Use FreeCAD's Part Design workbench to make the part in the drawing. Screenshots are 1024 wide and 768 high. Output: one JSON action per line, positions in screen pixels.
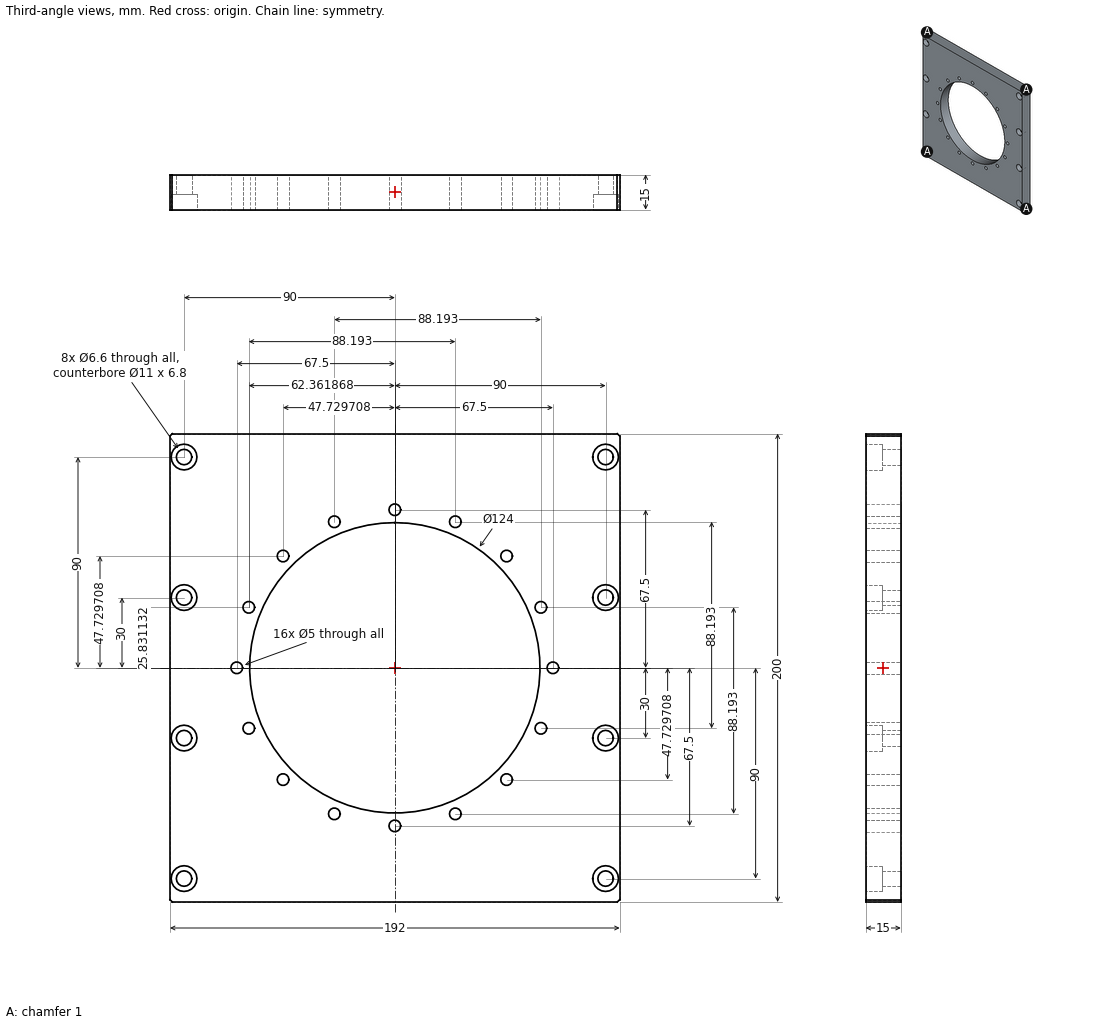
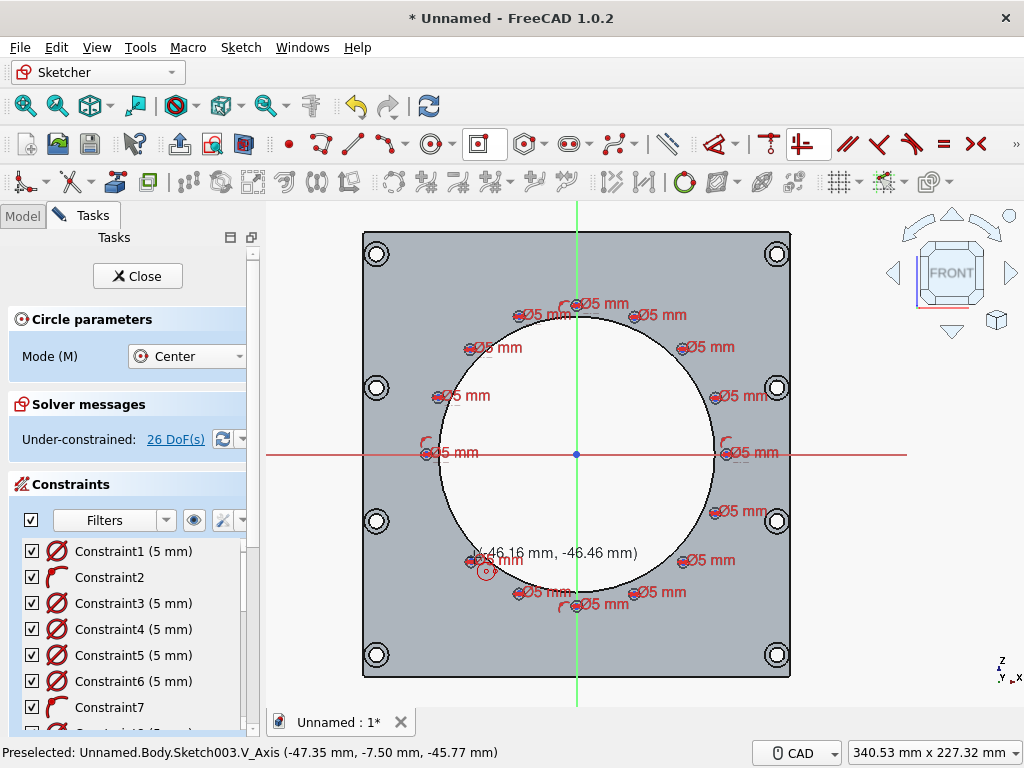
{"action": "scroll", "coordinate": [438, 512], "scroll_direction": "up", "scroll_amount": 8}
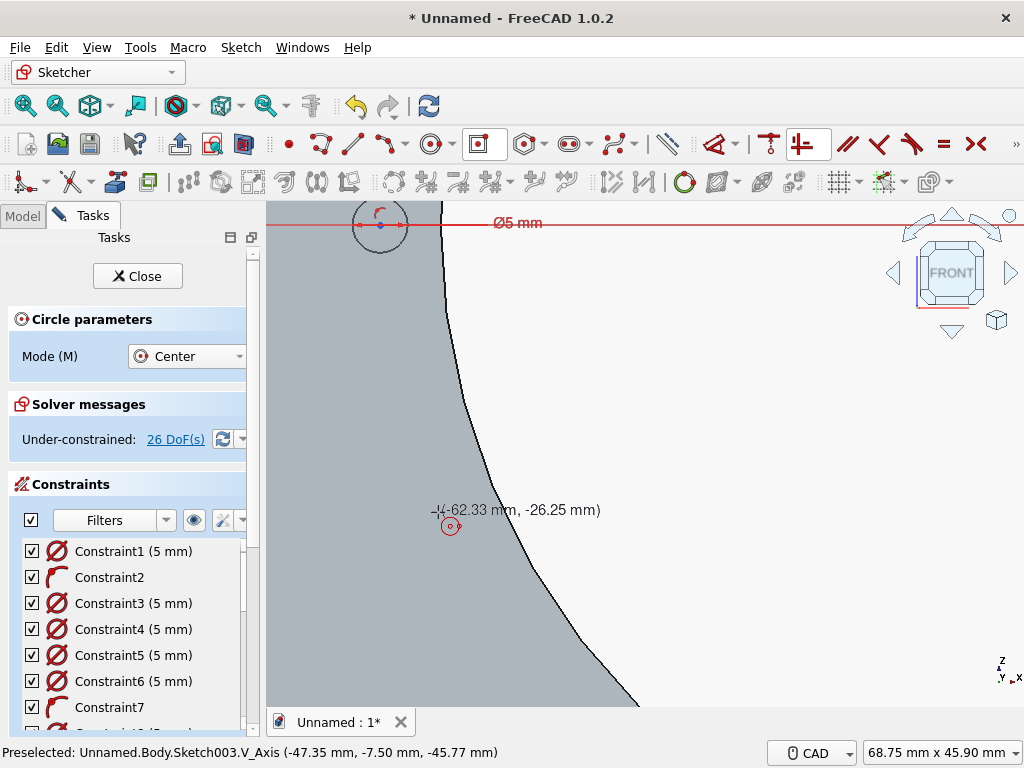
{"action": "scroll", "coordinate": [438, 512], "scroll_direction": "down", "scroll_amount": 8}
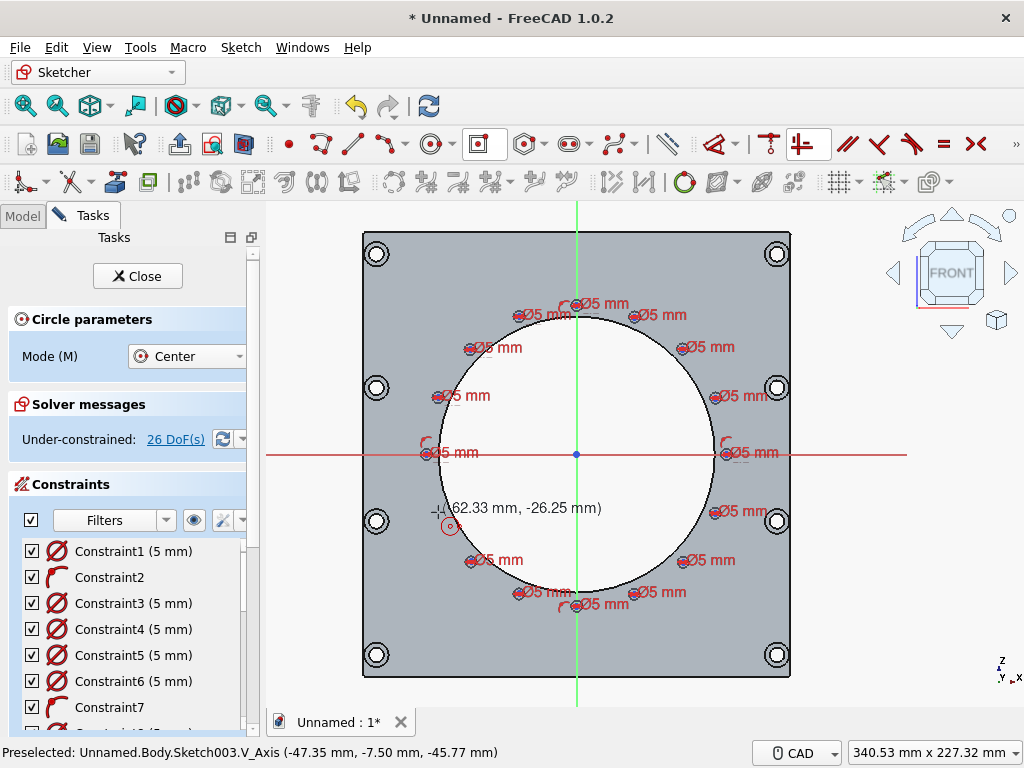
{"action": "left_click", "coordinate": [438, 512]}
{"action": "mouse_move", "coordinate": [442, 508]}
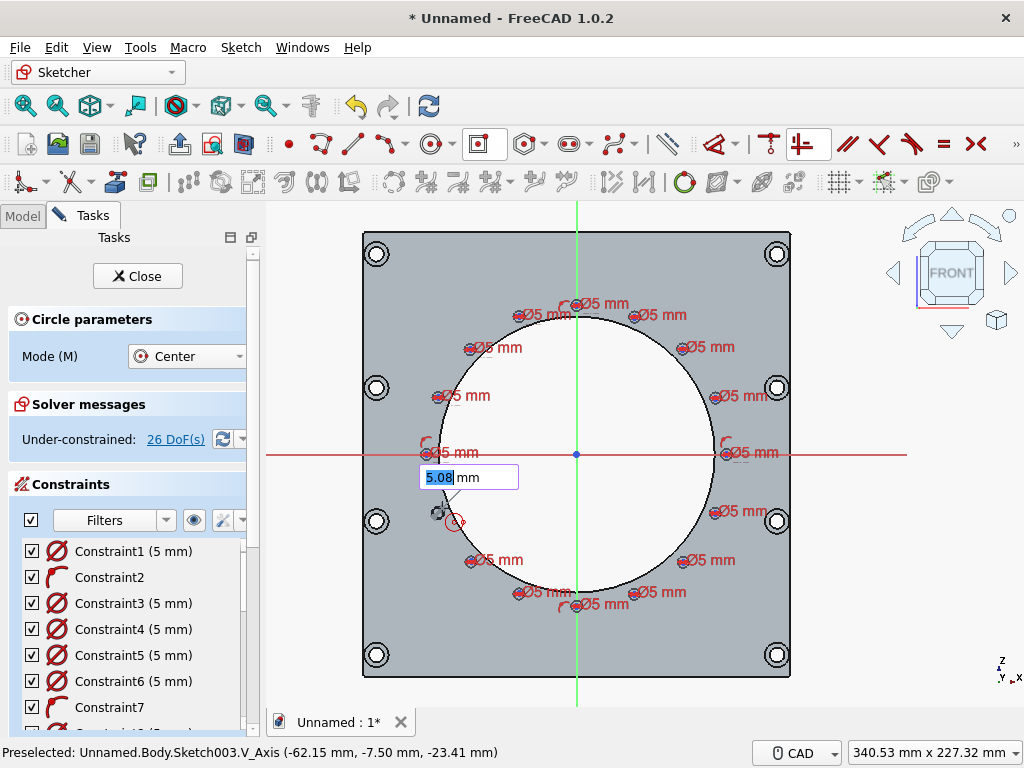
{"action": "type", "text": "5"}
{"action": "key", "text": "Return"}
{"action": "key", "text": "Escape"}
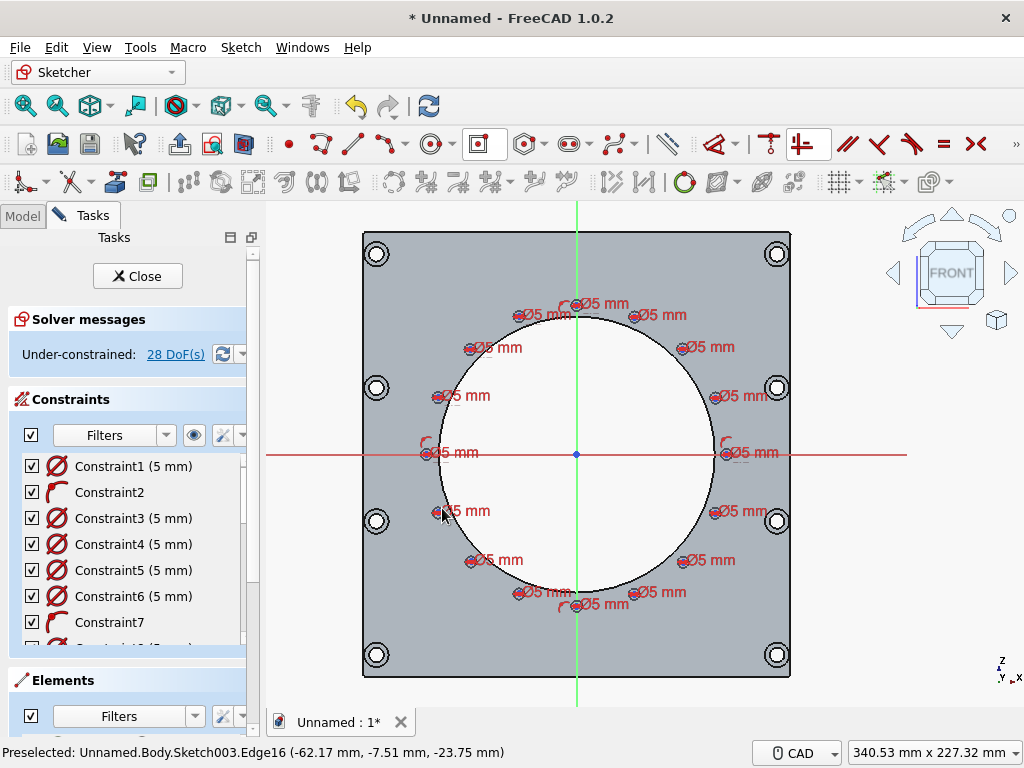
{"action": "left_click", "coordinate": [519, 317]}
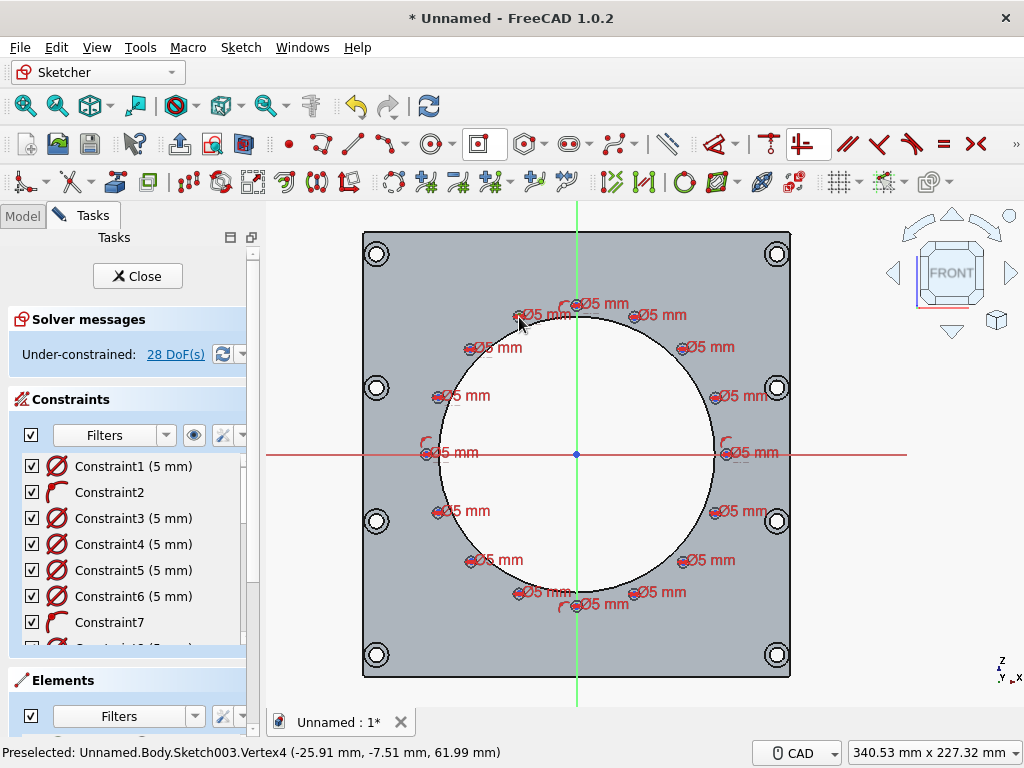
{"action": "left_click", "coordinate": [635, 317]}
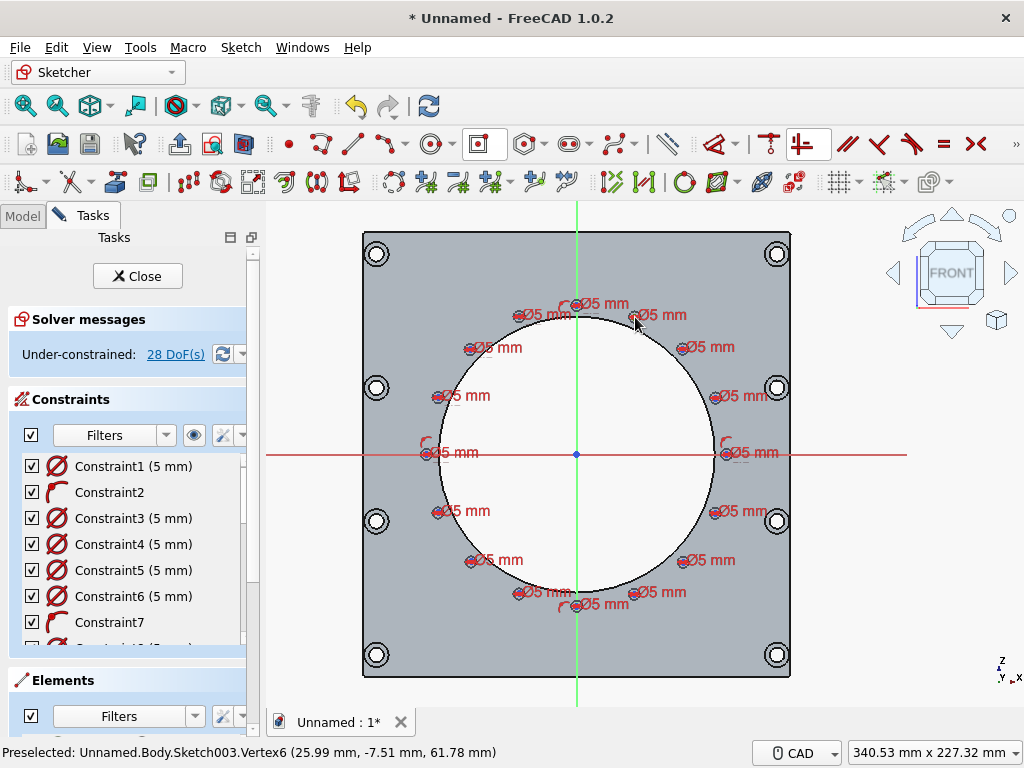
{"action": "key", "text": "h"}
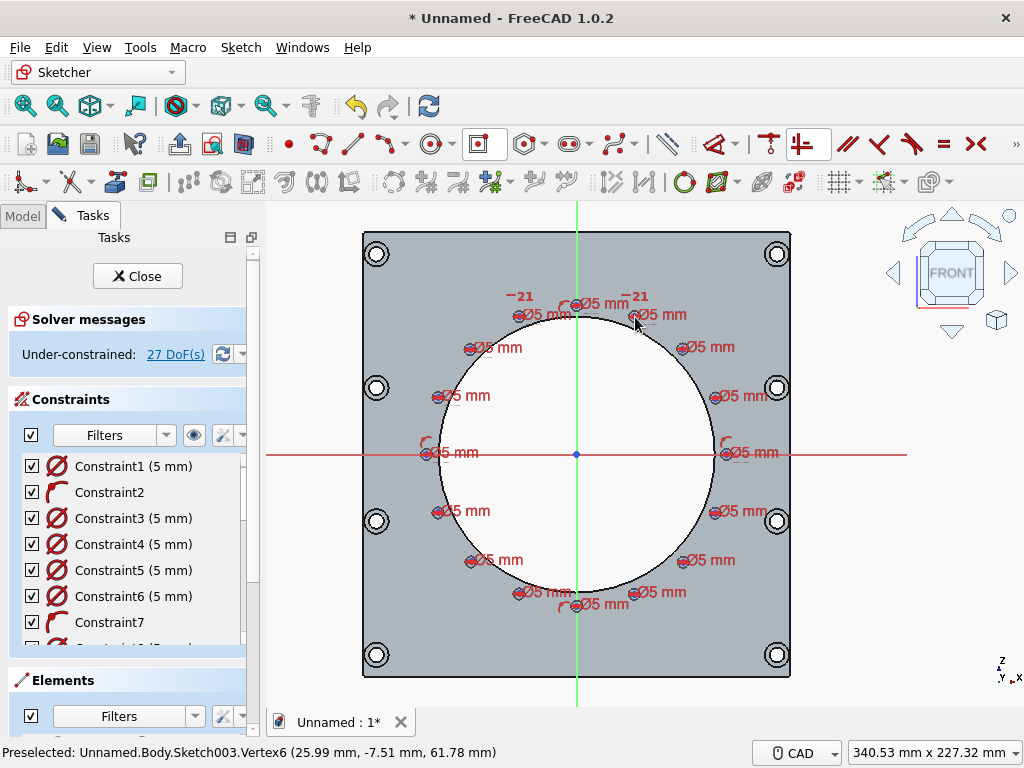
{"action": "left_click", "coordinate": [470, 350]}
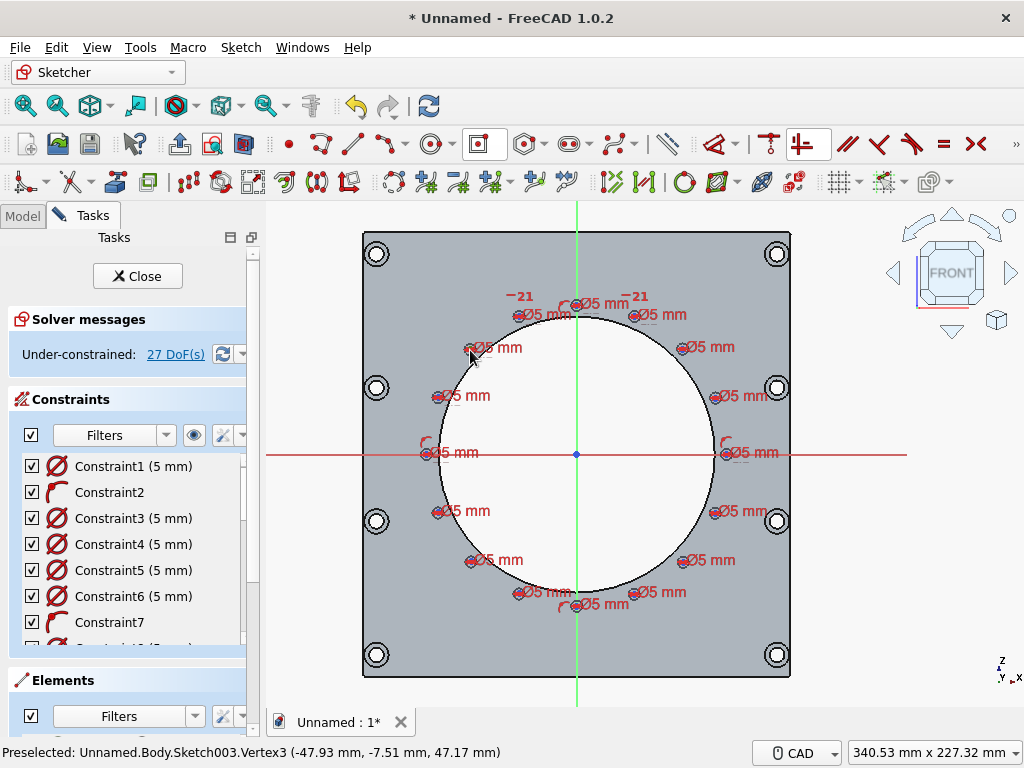
{"action": "left_click", "coordinate": [683, 349]}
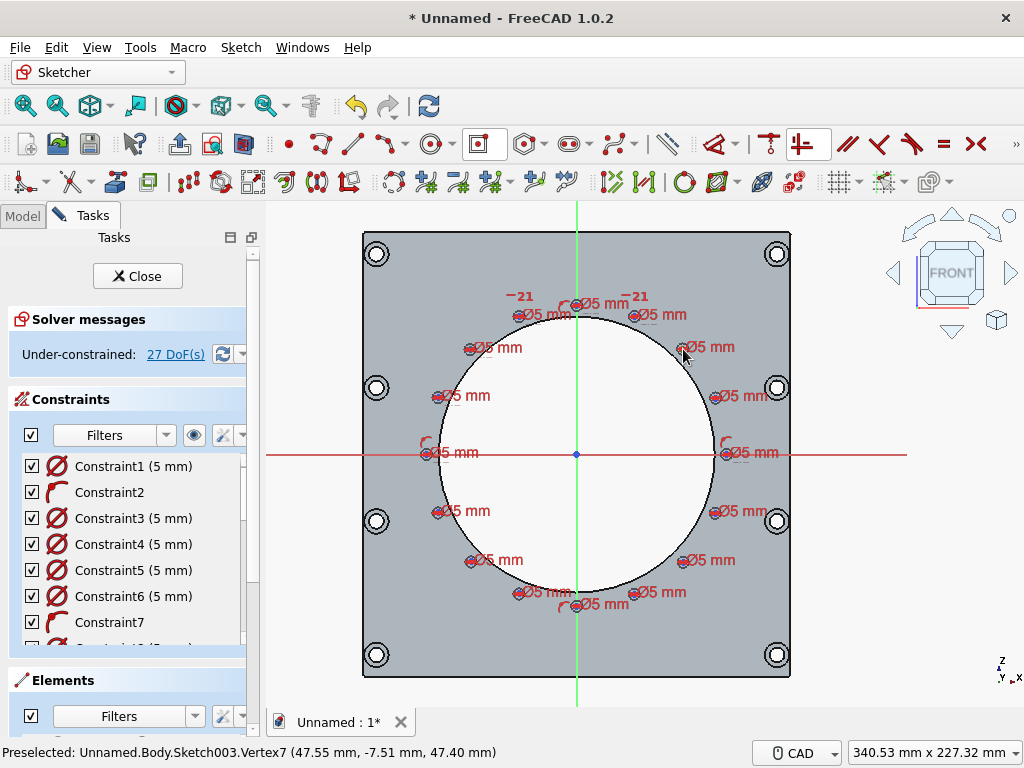
{"action": "key", "text": "h"}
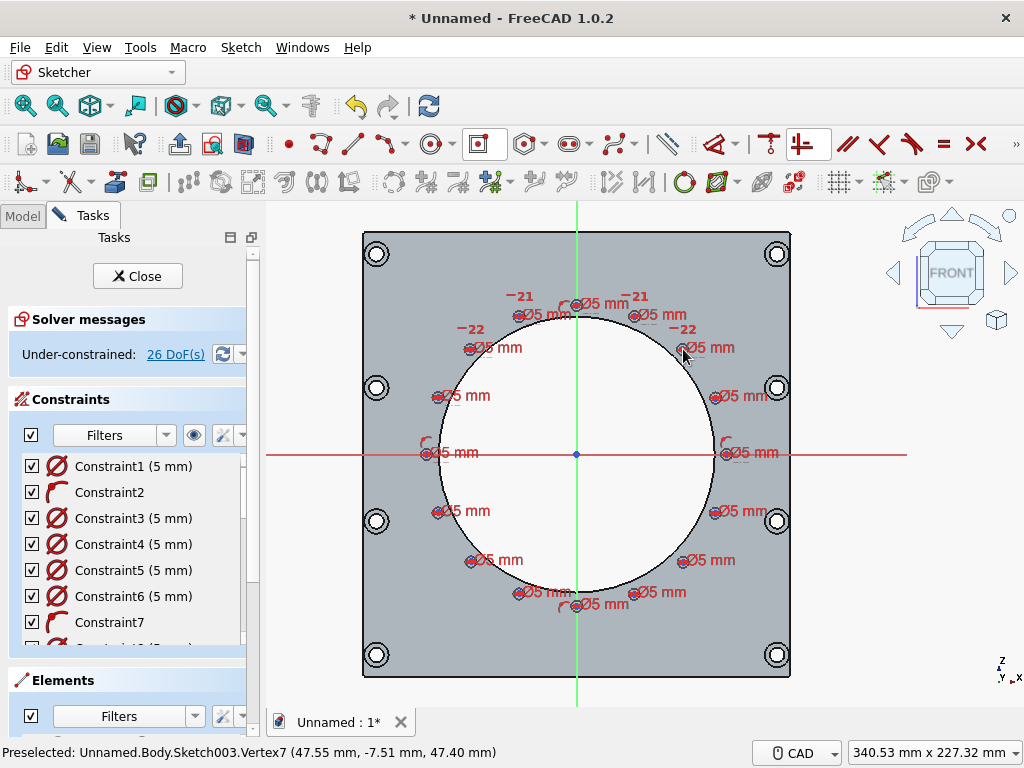
{"action": "left_click", "coordinate": [438, 398]}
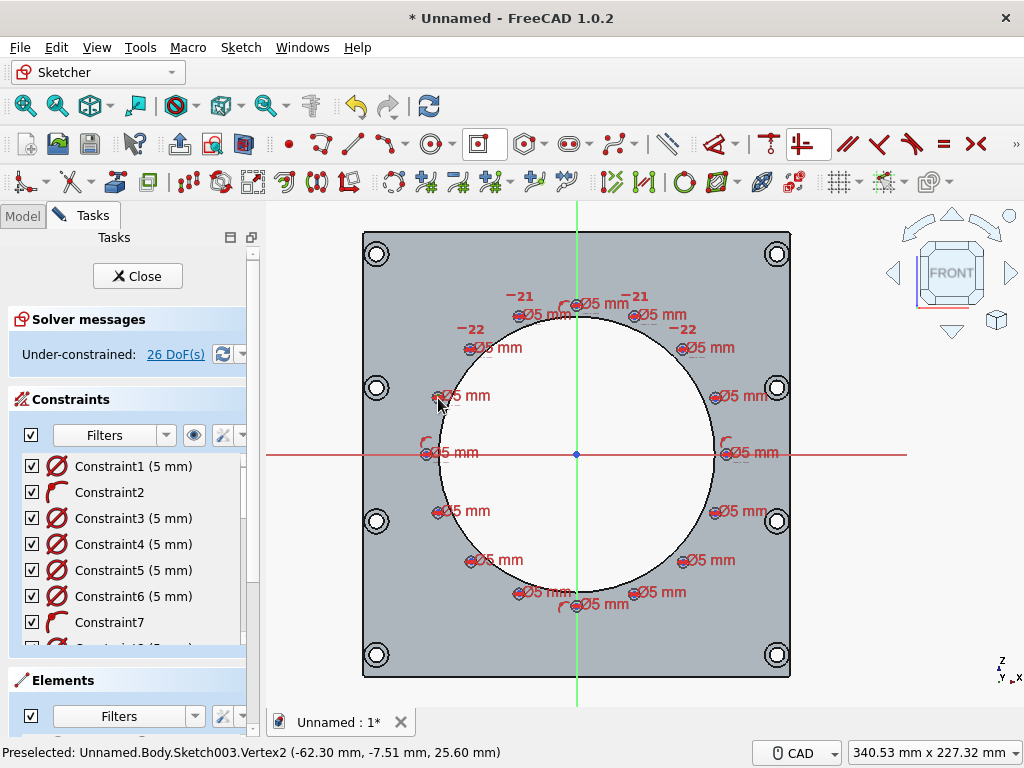
{"action": "left_click", "coordinate": [716, 398]}